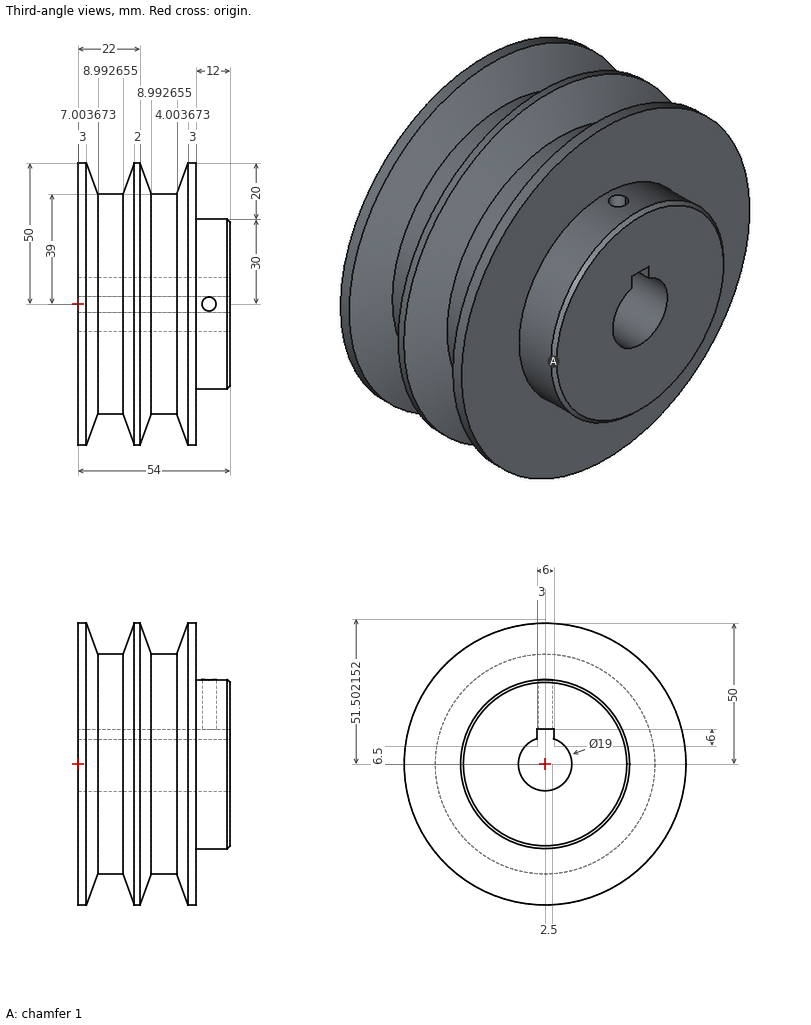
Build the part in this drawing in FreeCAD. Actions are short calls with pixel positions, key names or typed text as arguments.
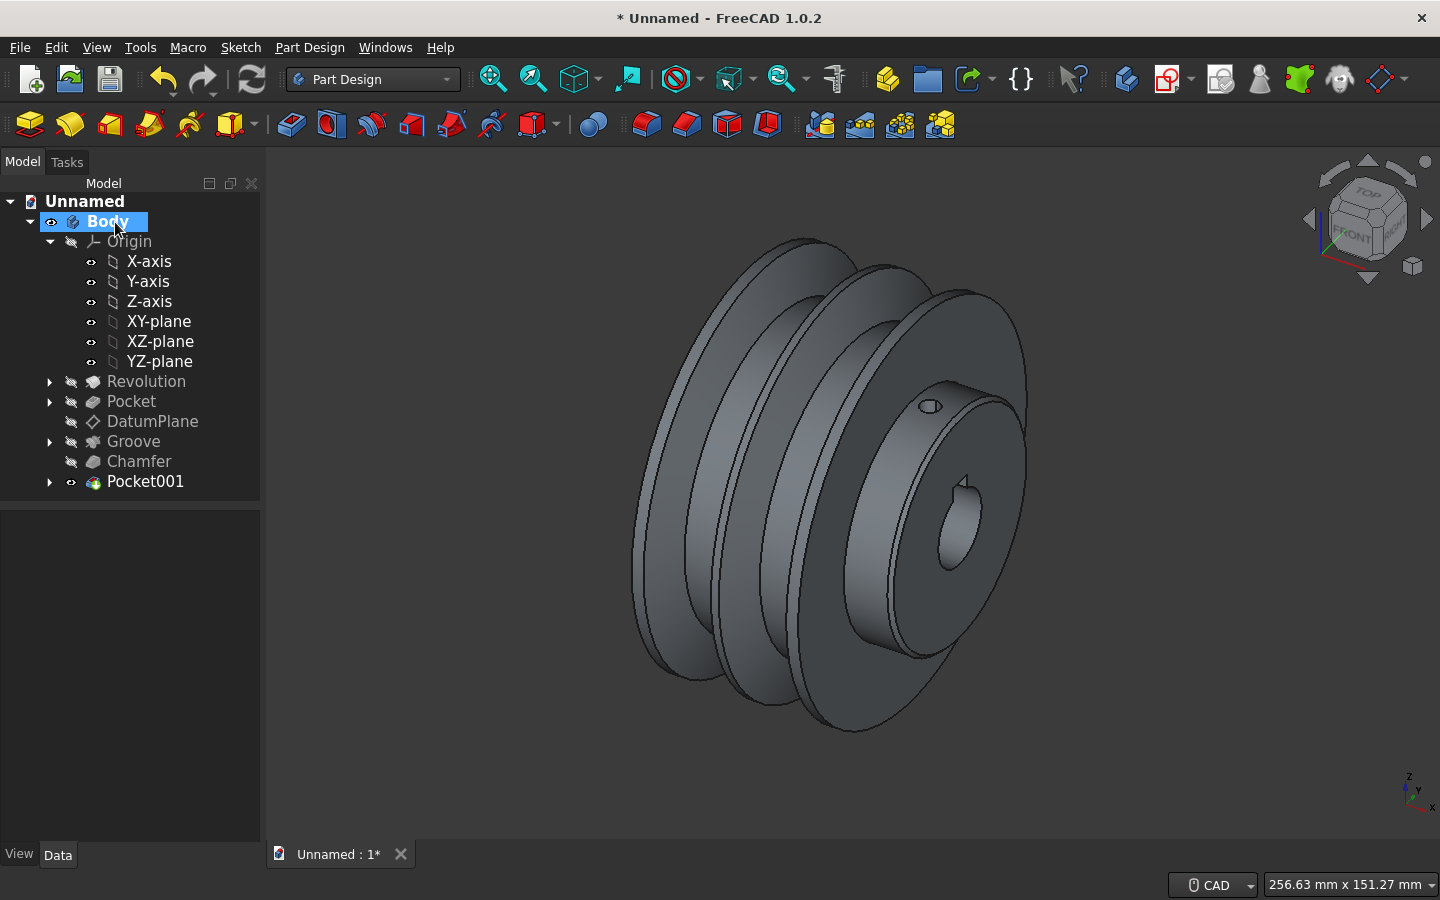
key(0)